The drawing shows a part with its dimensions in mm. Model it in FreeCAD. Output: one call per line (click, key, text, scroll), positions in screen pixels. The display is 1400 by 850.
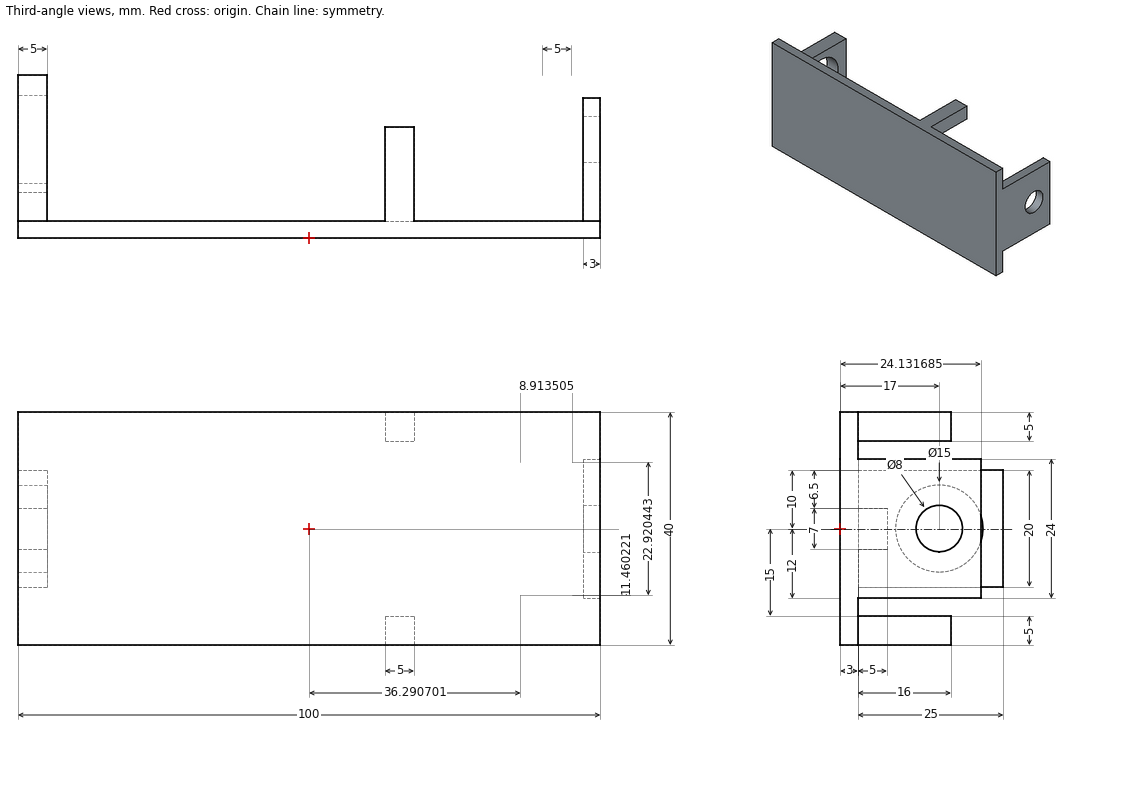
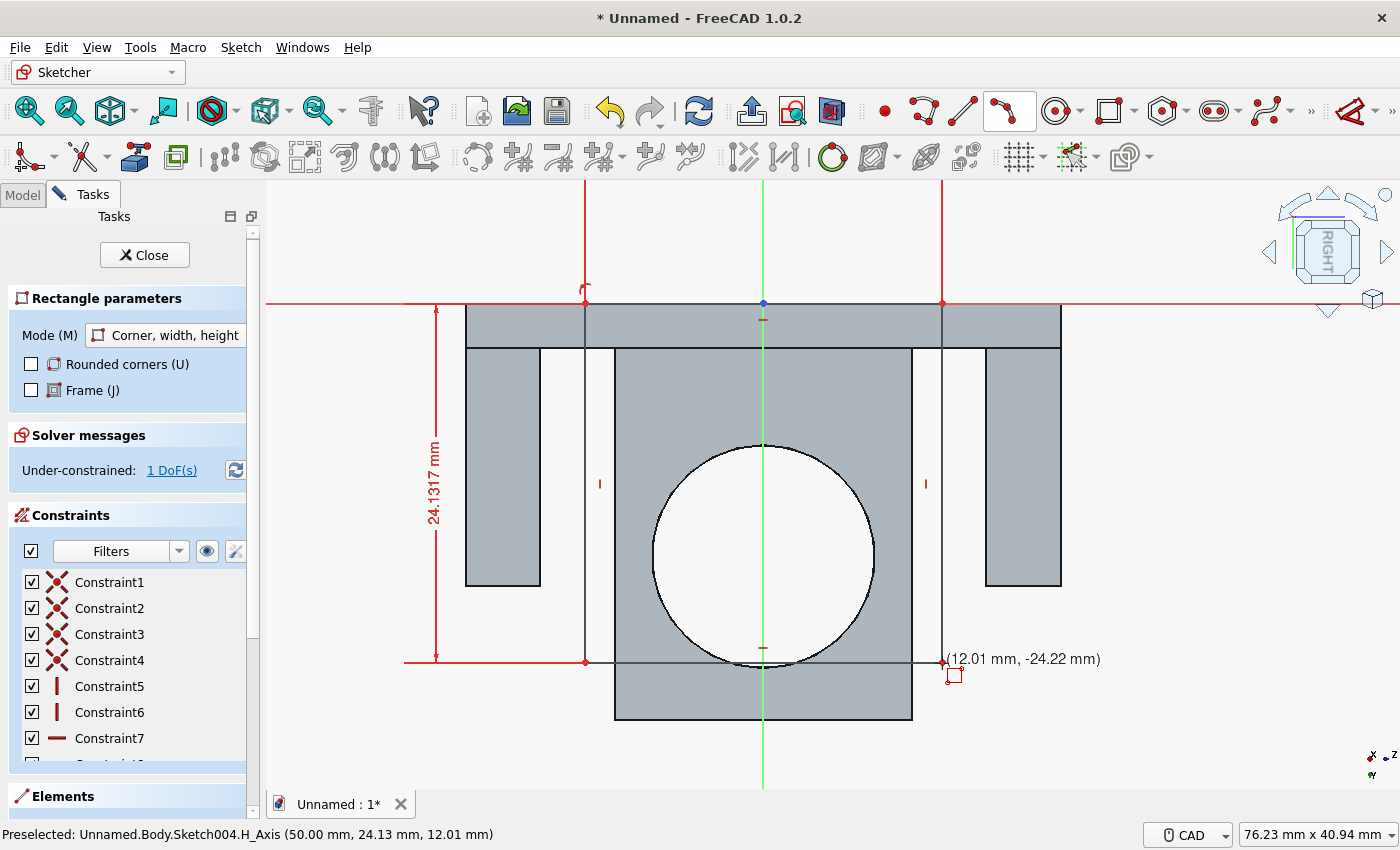
click(1056, 112)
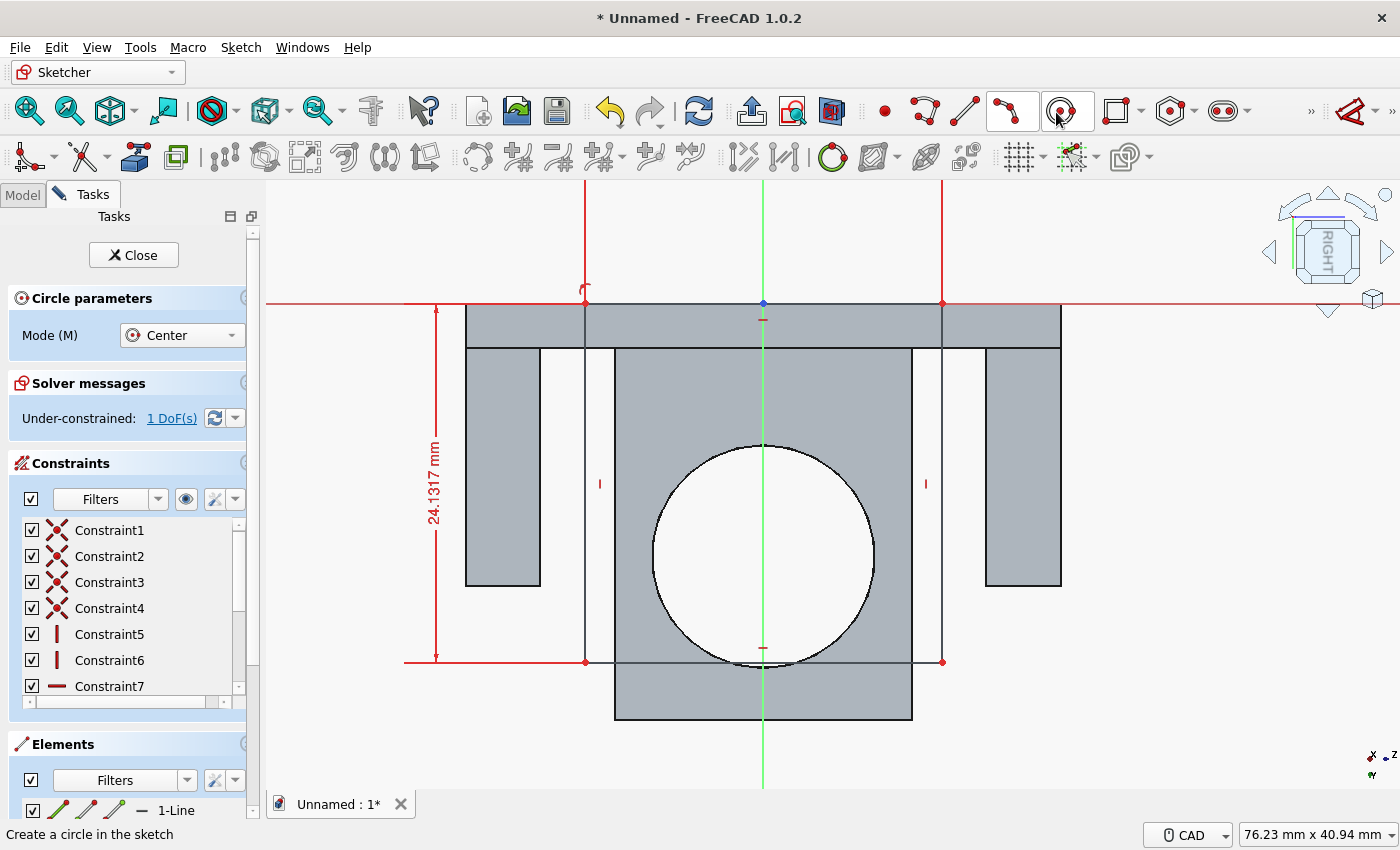
click(763, 557)
move(805, 515)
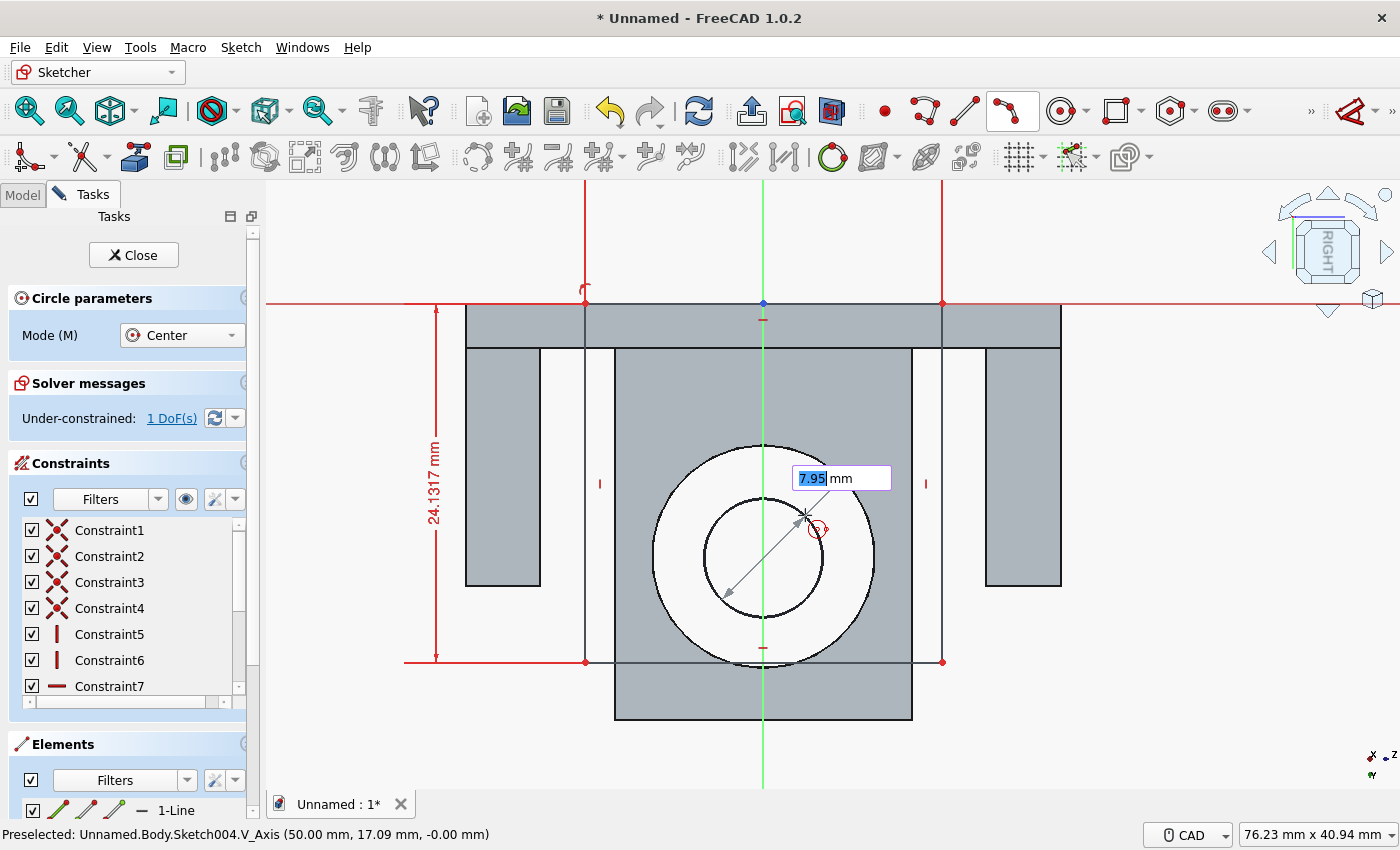
text(8)
key(Return)
key(Escape)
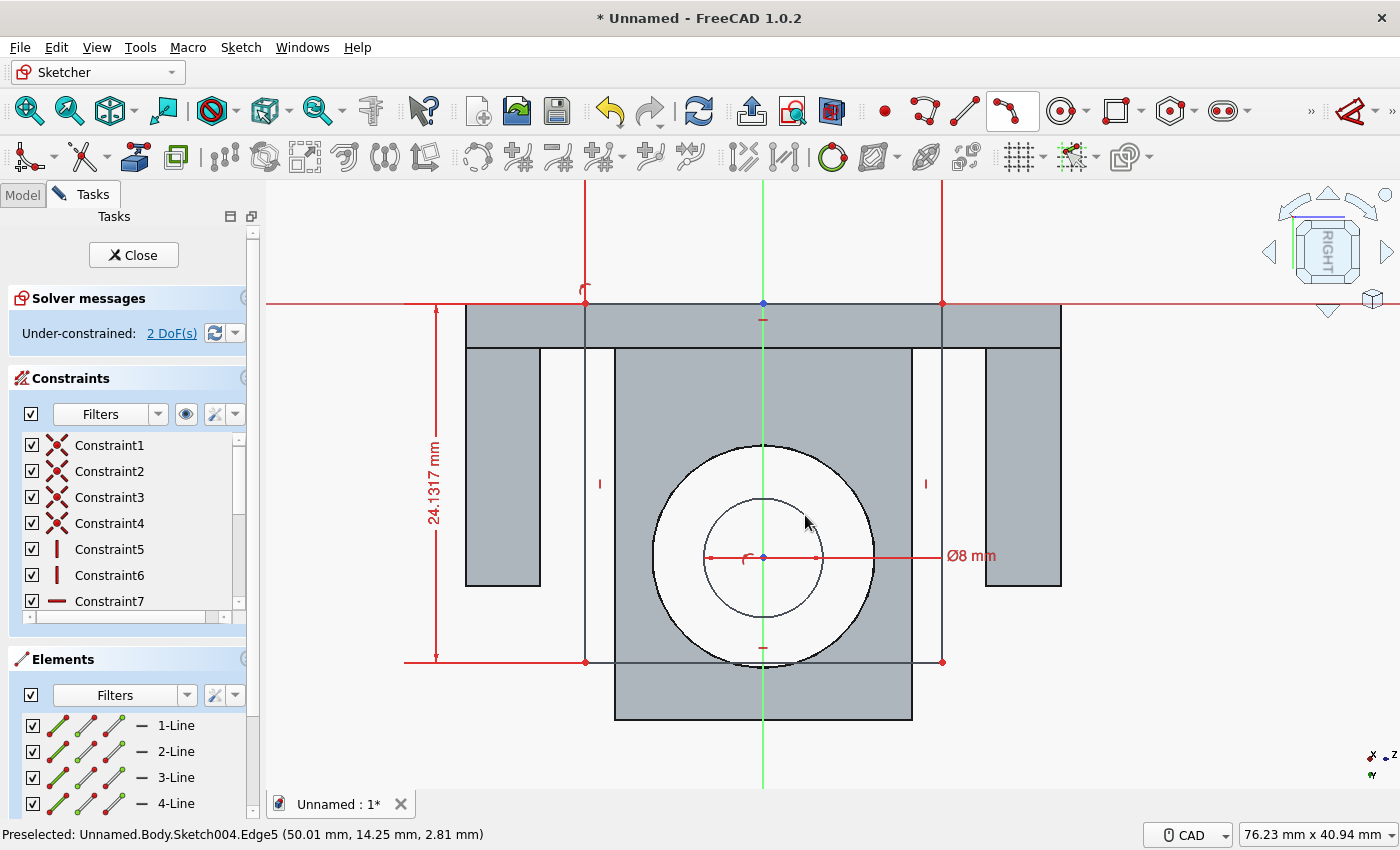
click(1350, 112)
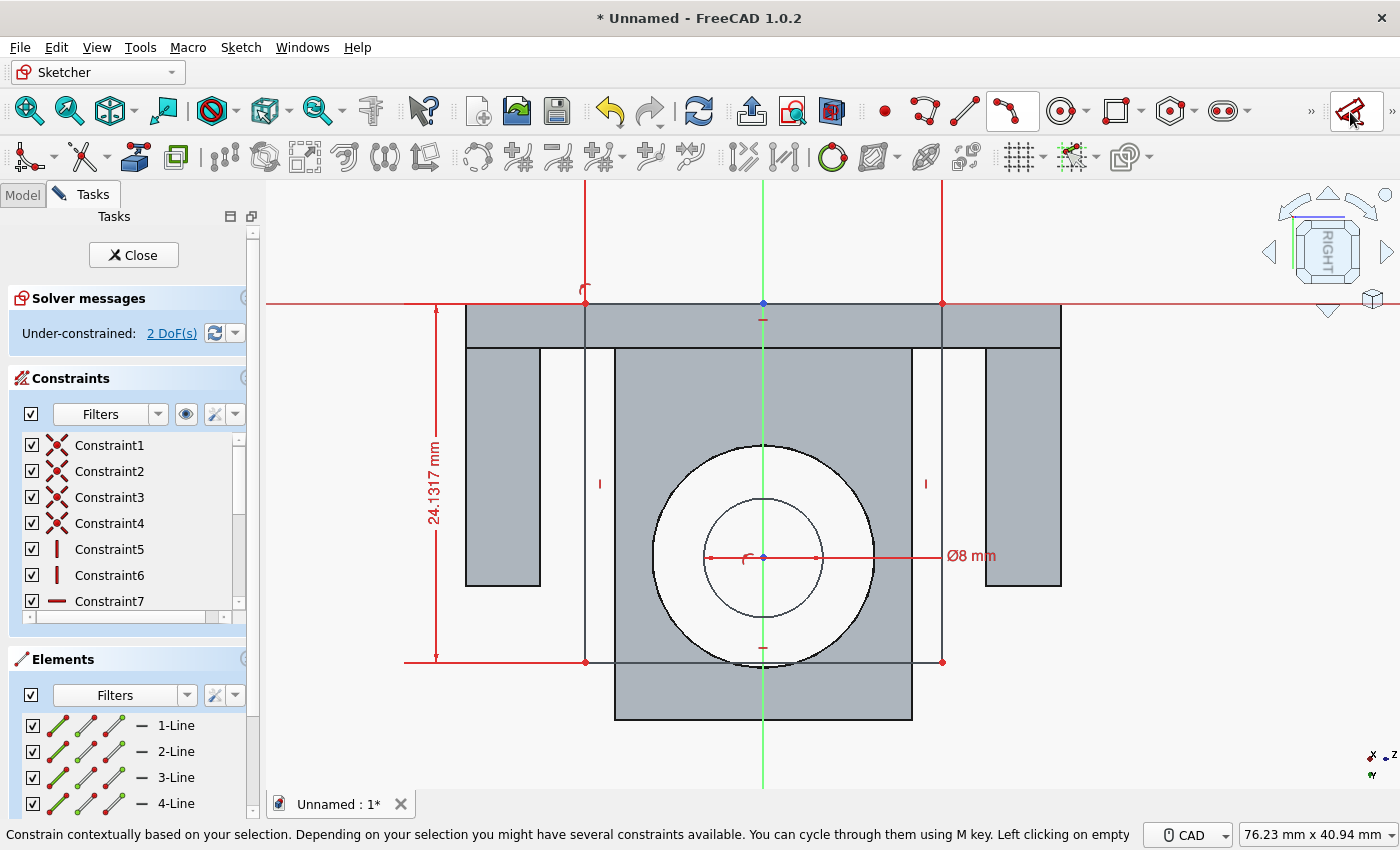
click(763, 558)
click(797, 431)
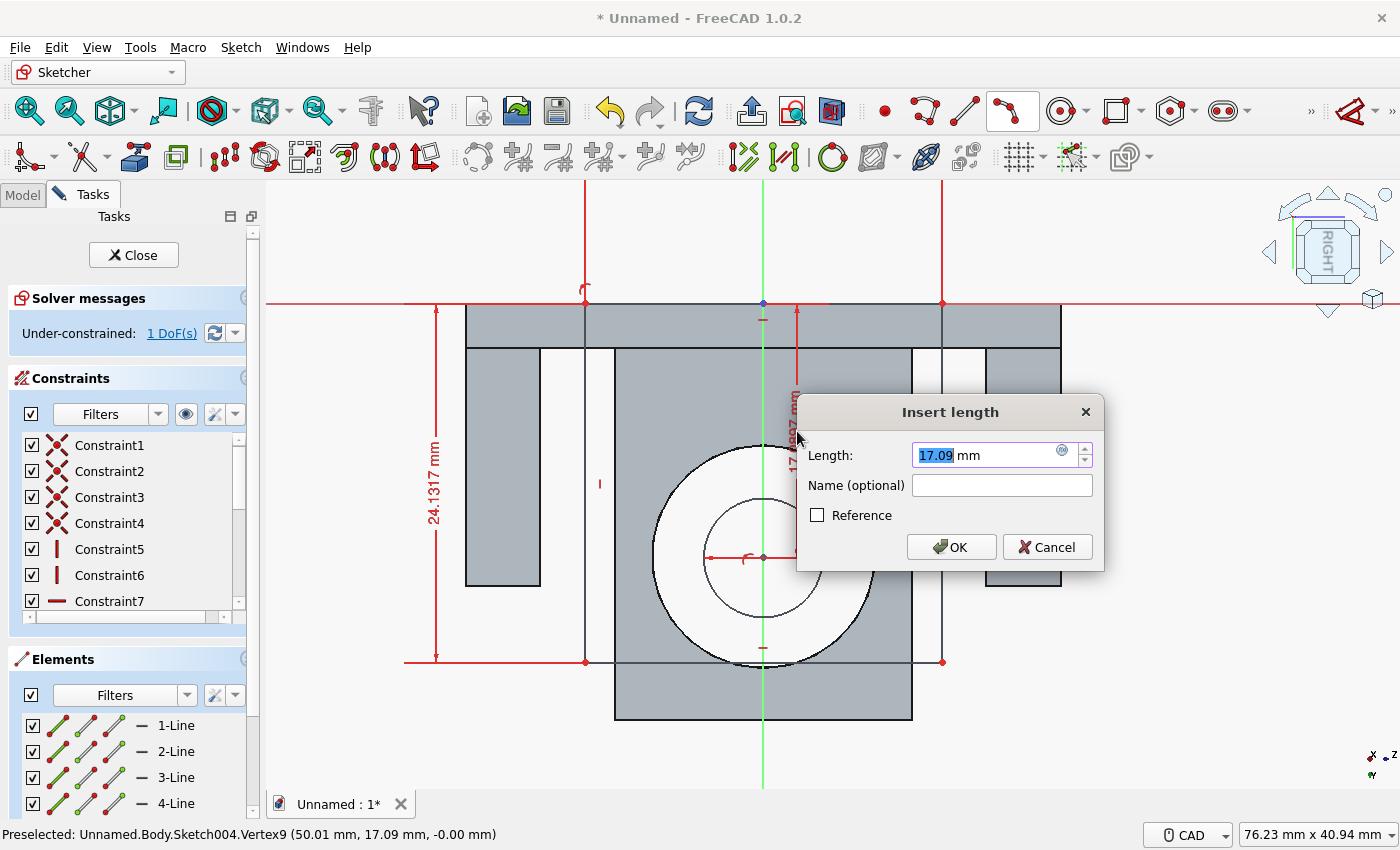
text(17)
key(Return)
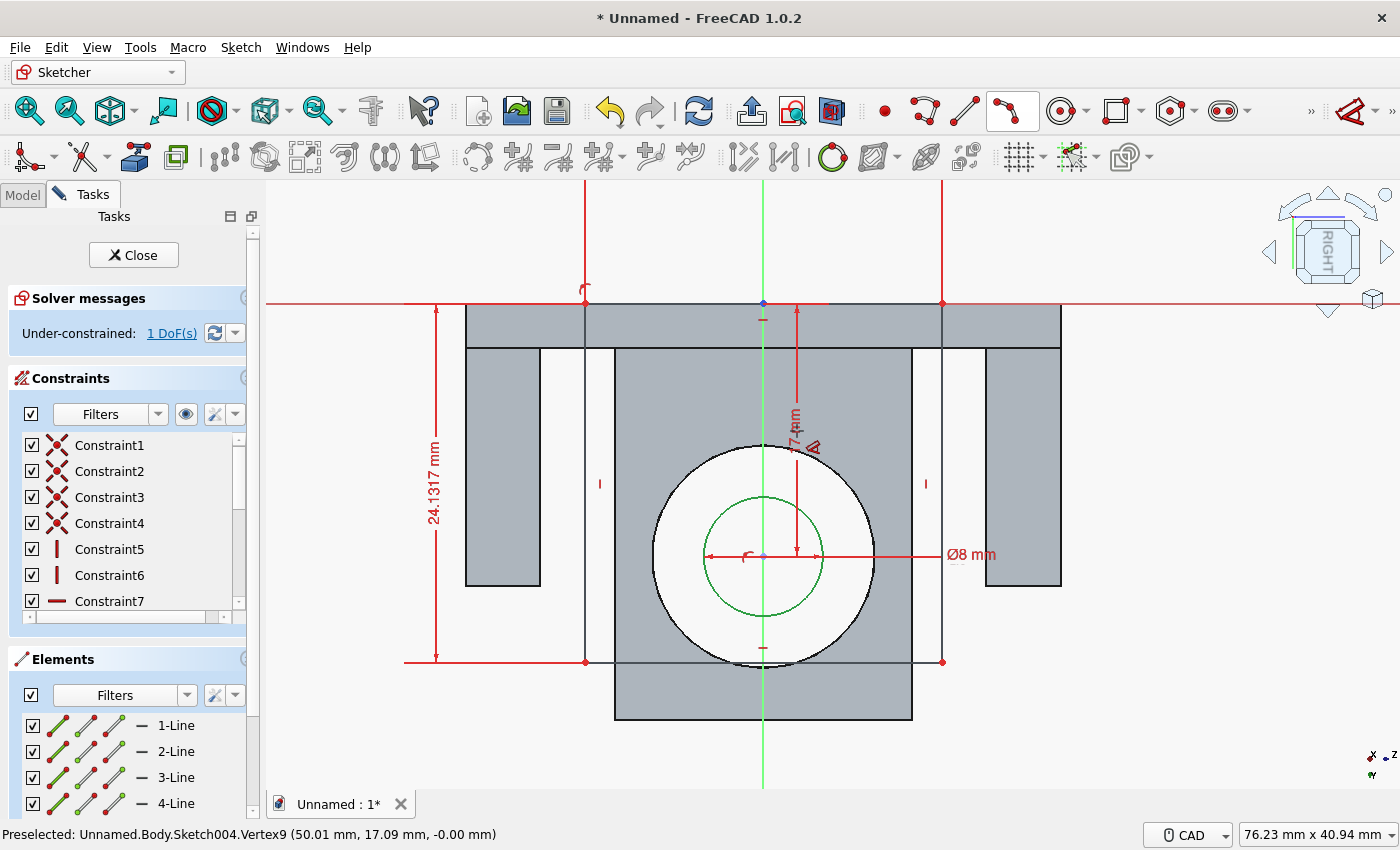
click(585, 304)
click(674, 270)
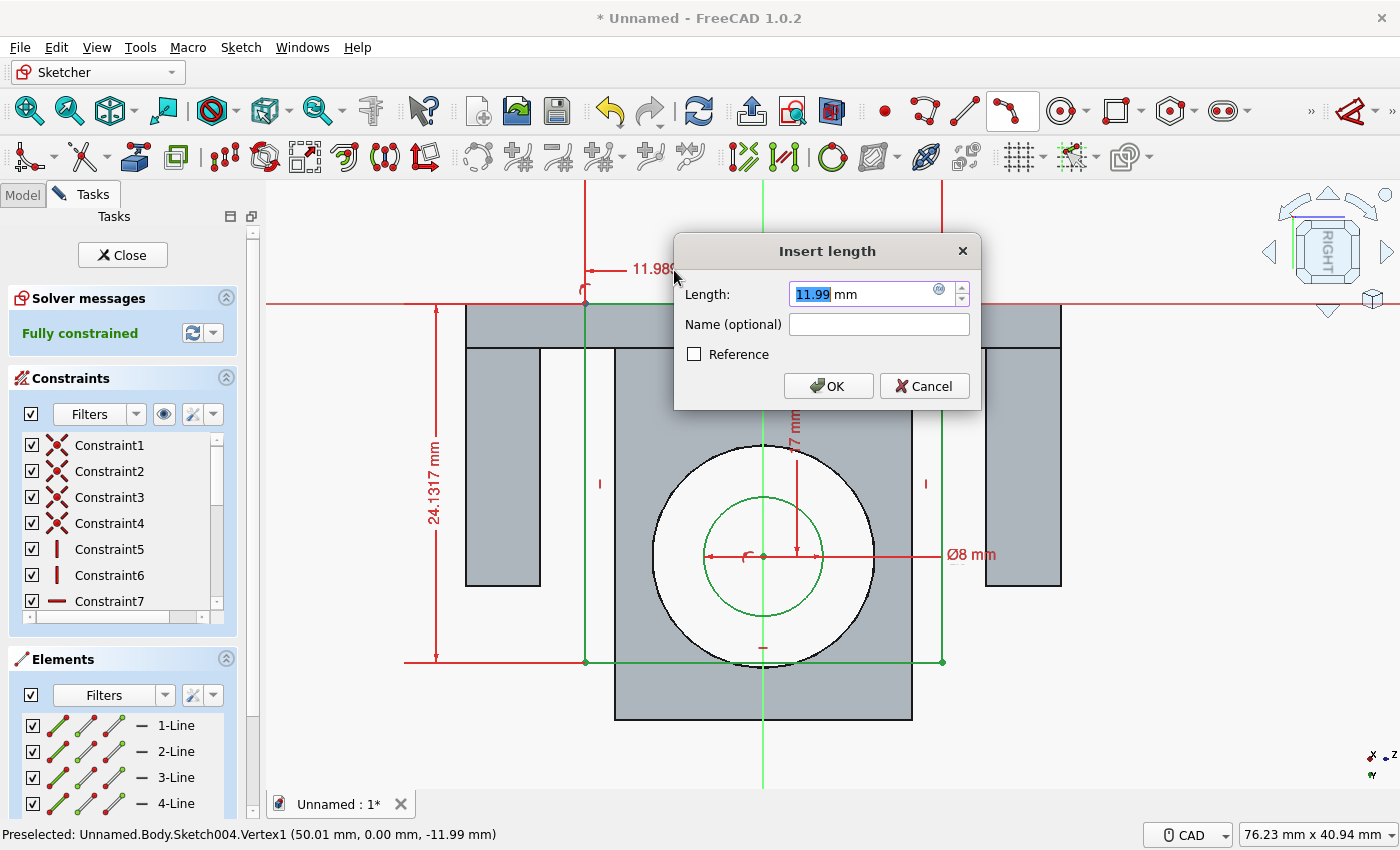
text(12)
key(Return)
key(Escape)